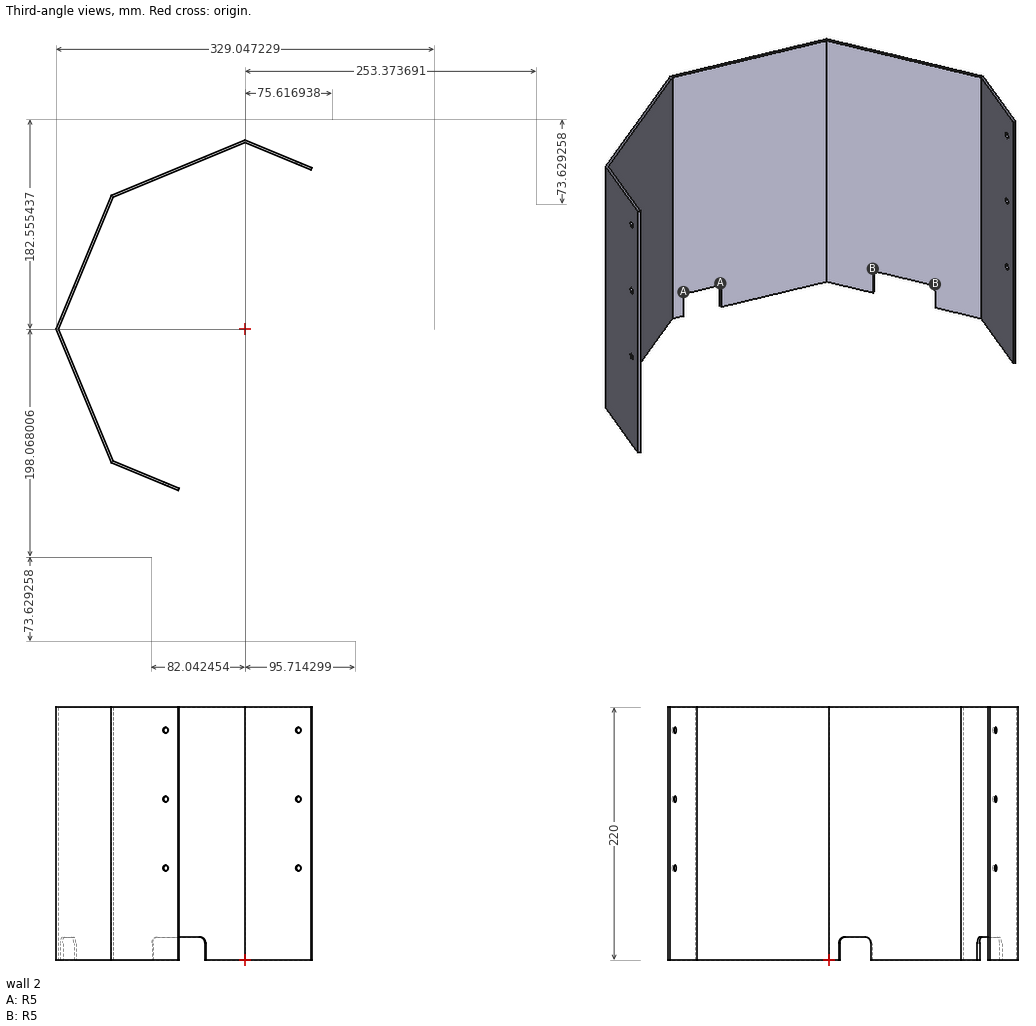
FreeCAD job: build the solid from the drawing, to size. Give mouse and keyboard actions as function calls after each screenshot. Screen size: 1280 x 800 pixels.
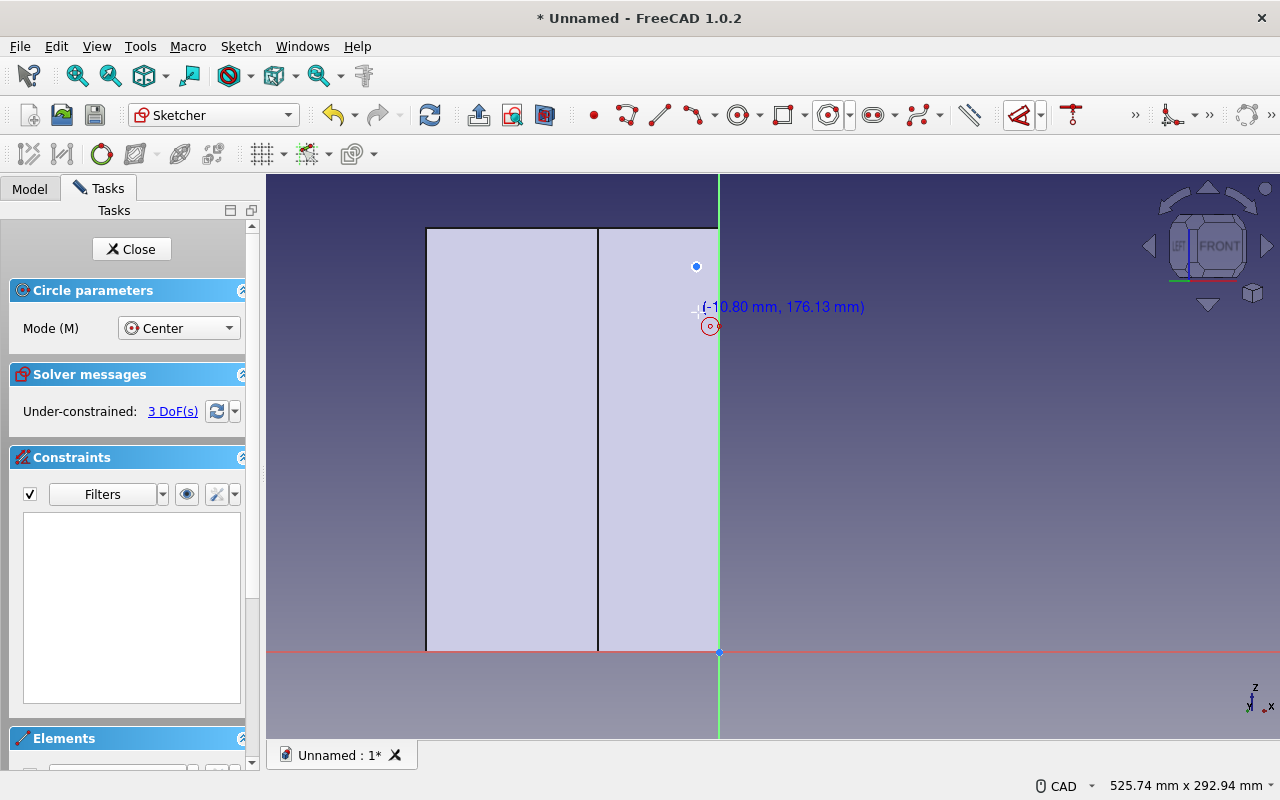
click(696, 382)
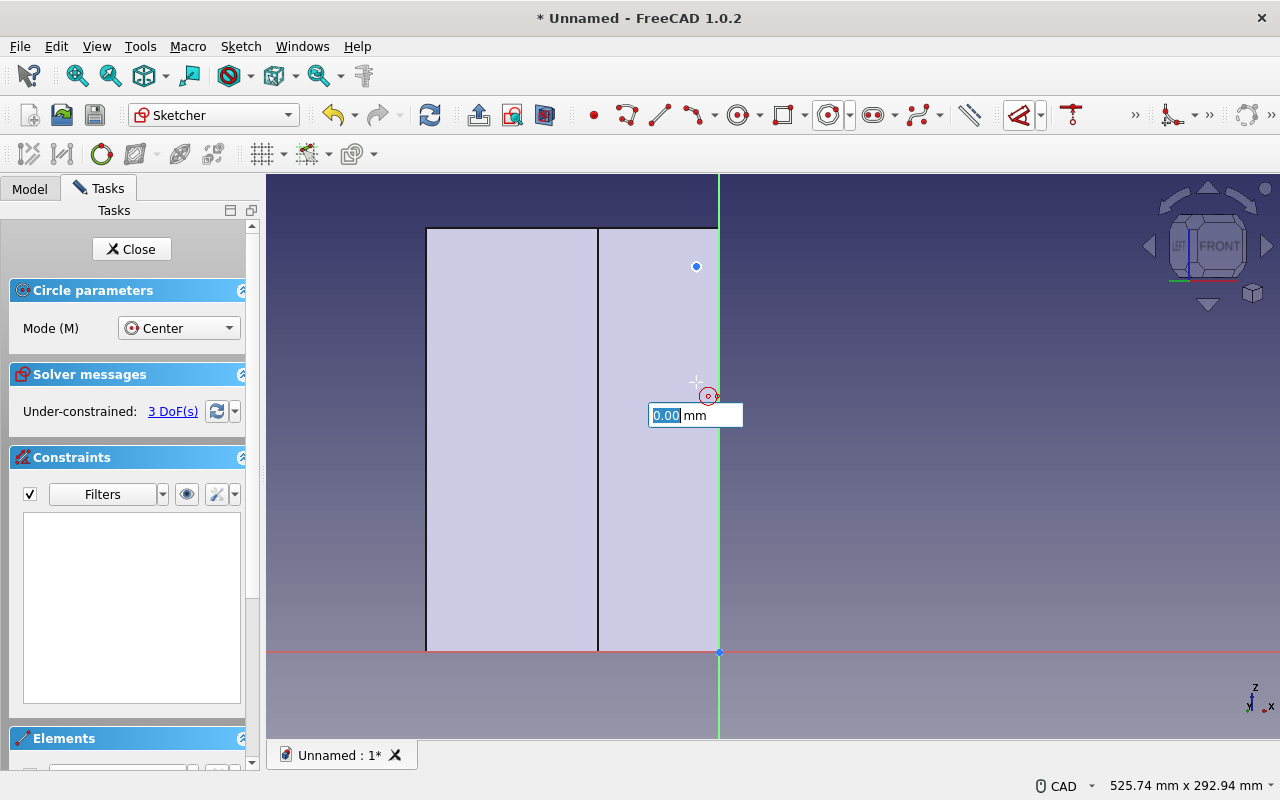
scroll(699, 379, up, 6)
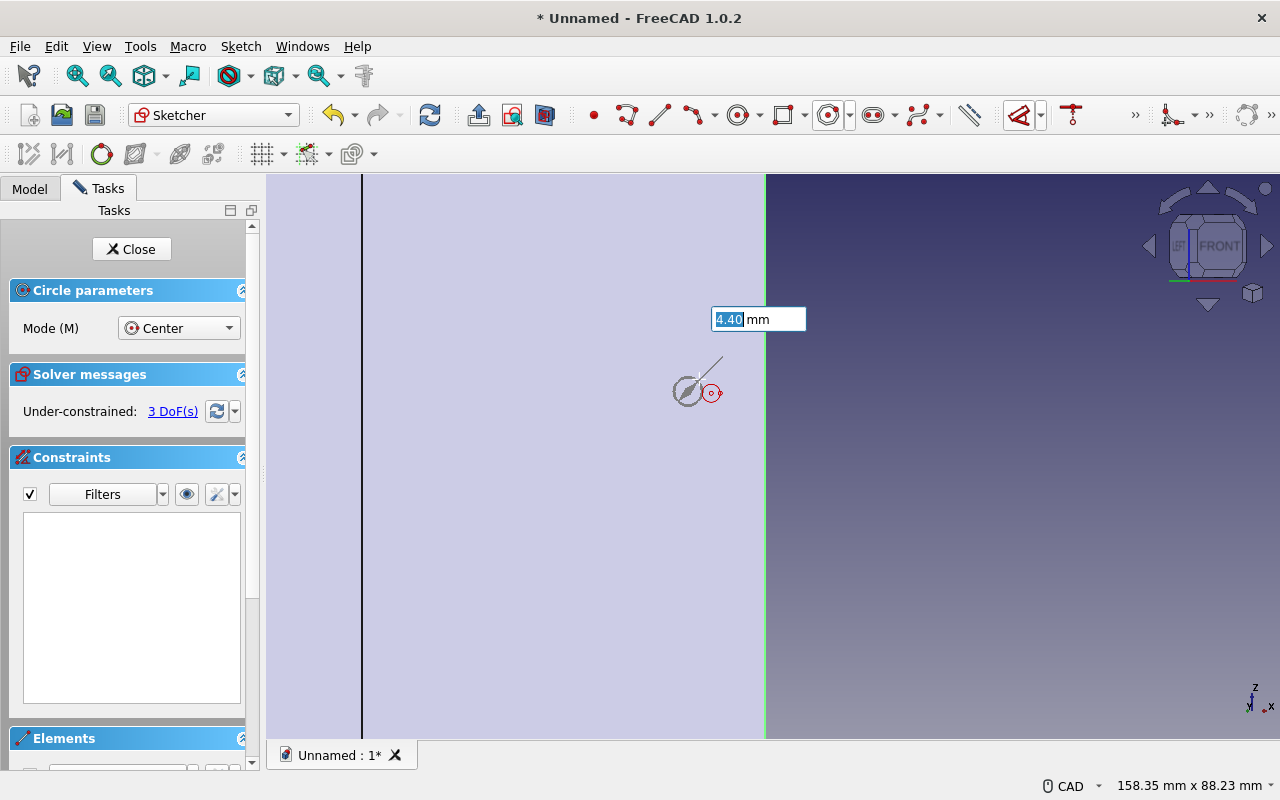
click(699, 377)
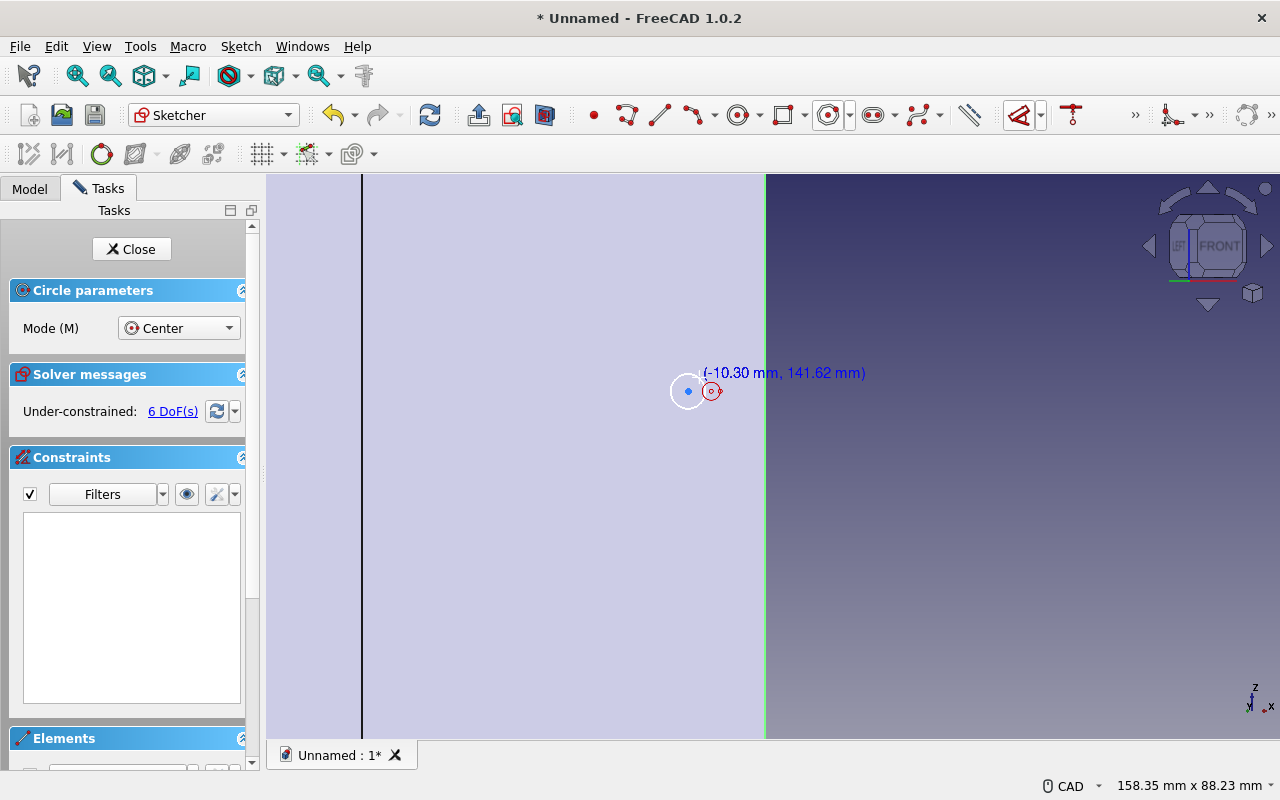
scroll(698, 379, down, 6)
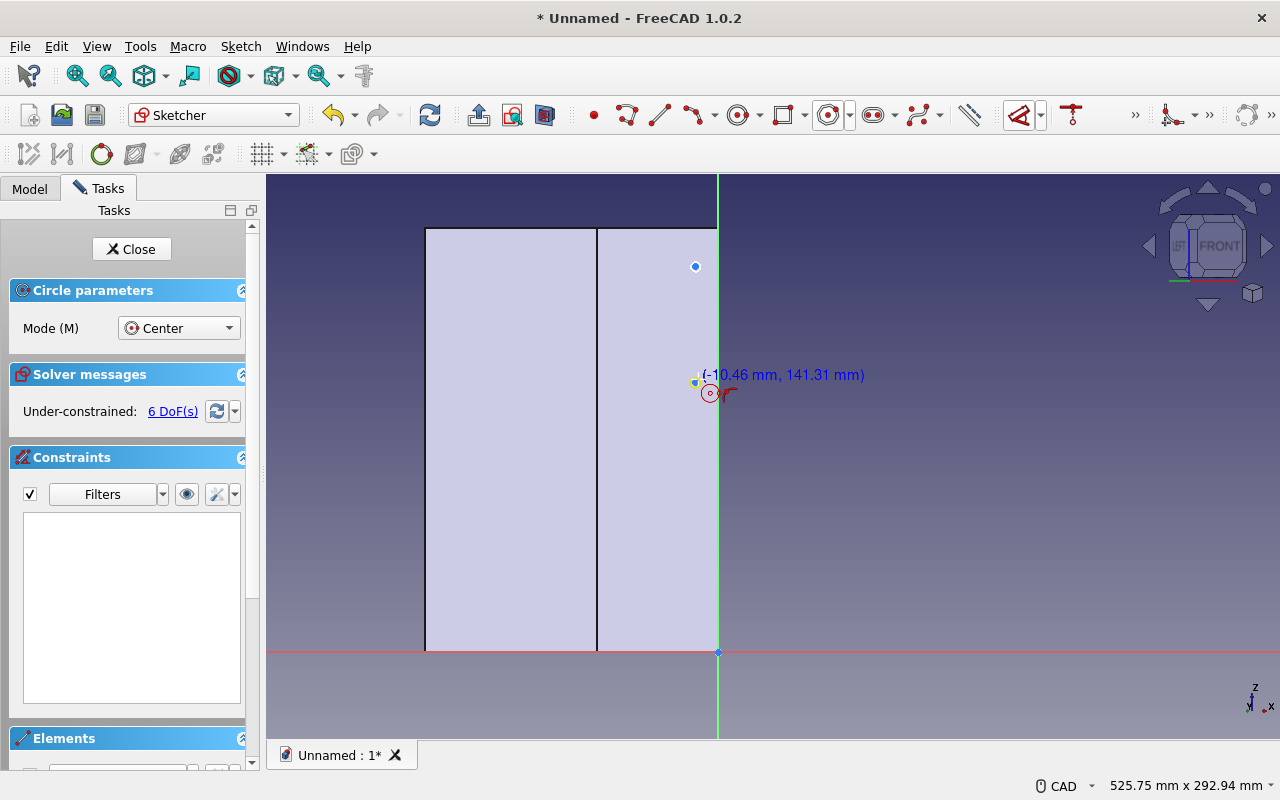
scroll(695, 498, up, 8)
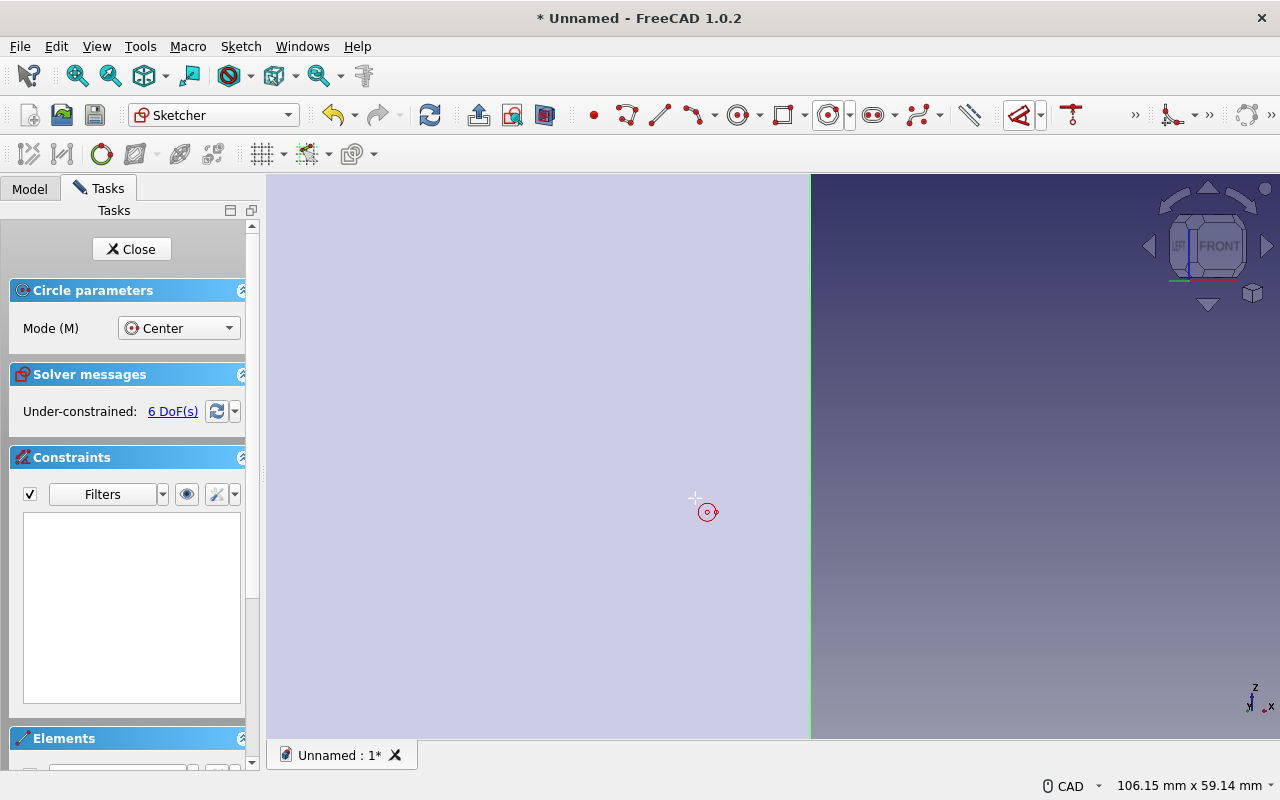
scroll(695, 498, down, 8)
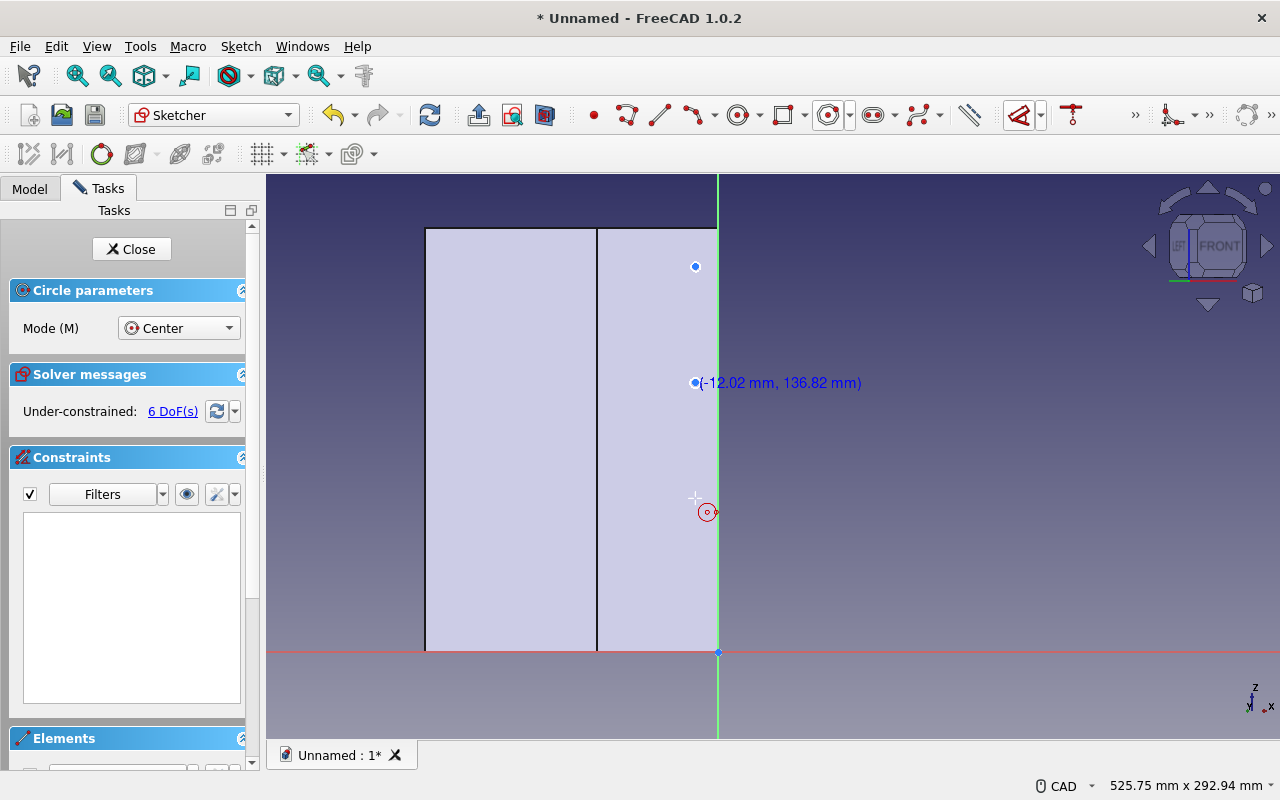
click(695, 498)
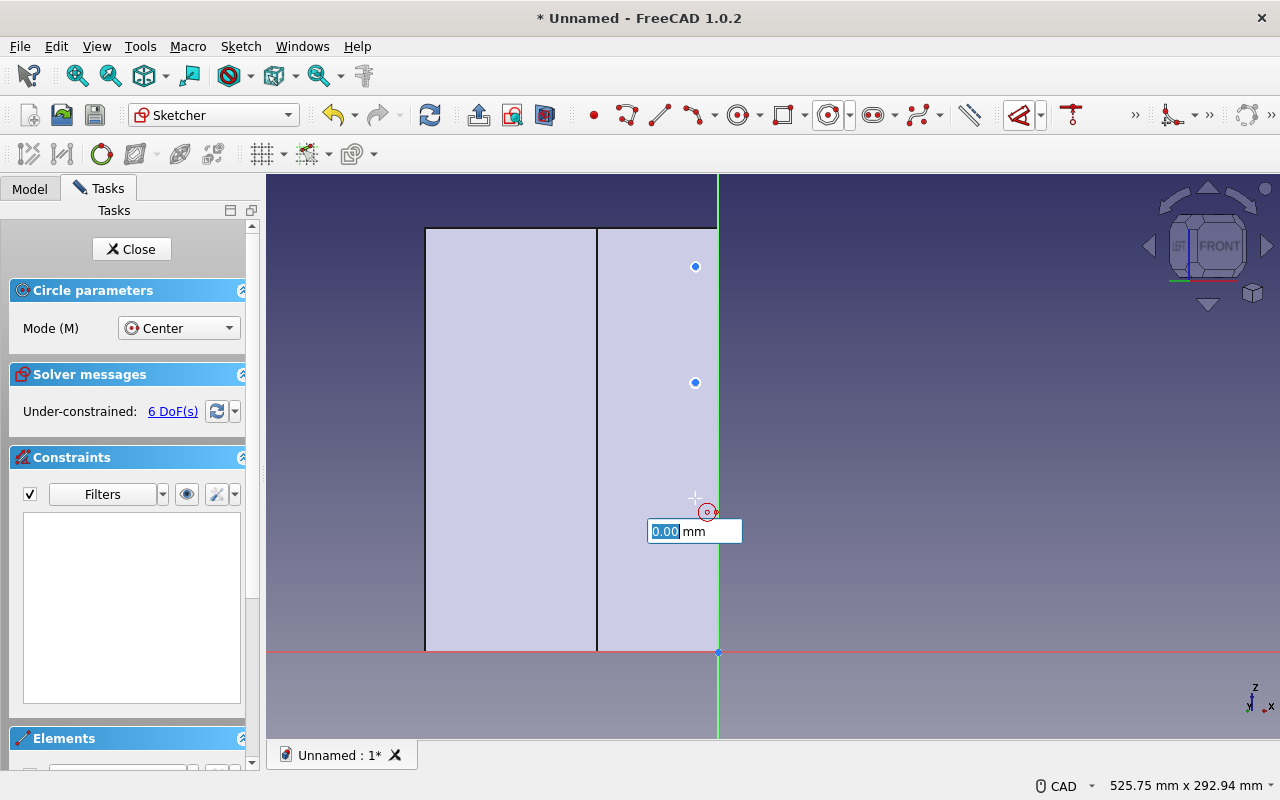
scroll(699, 494, up, 6)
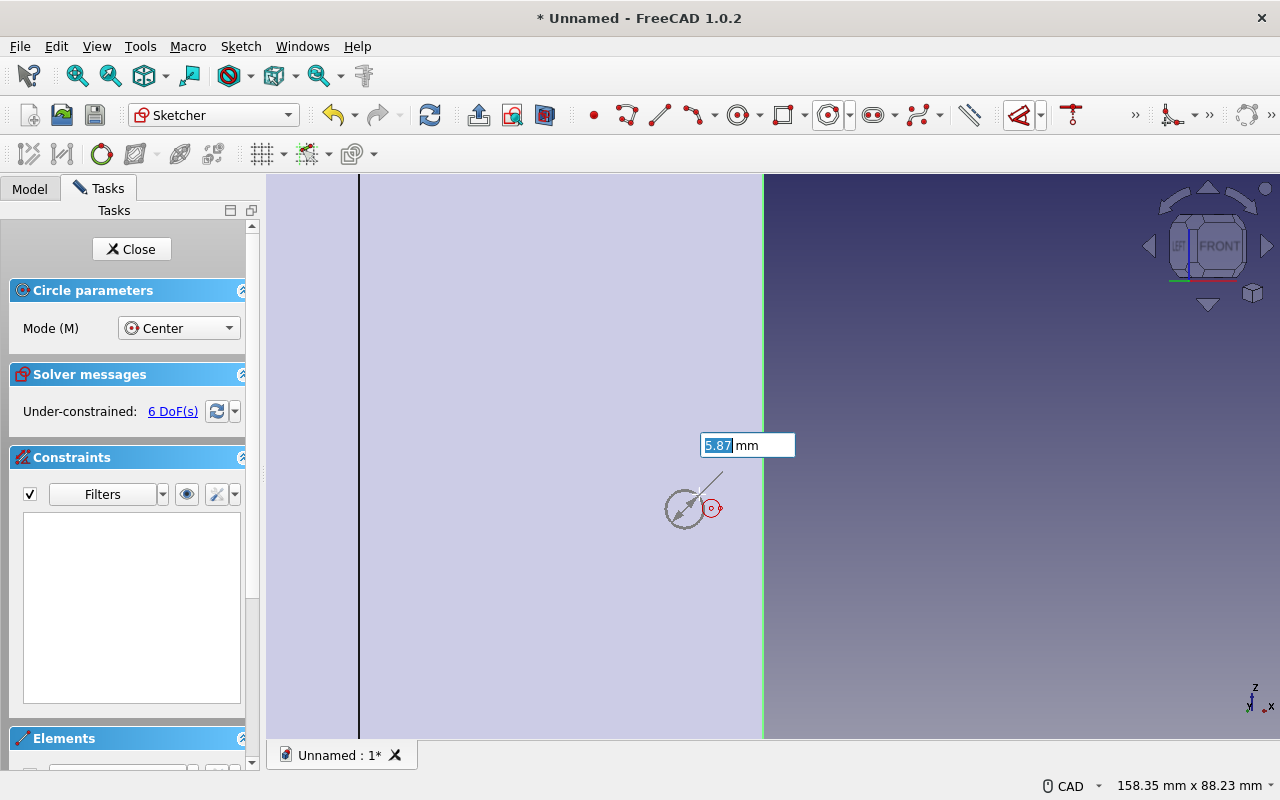
click(697, 494)
key(Escape)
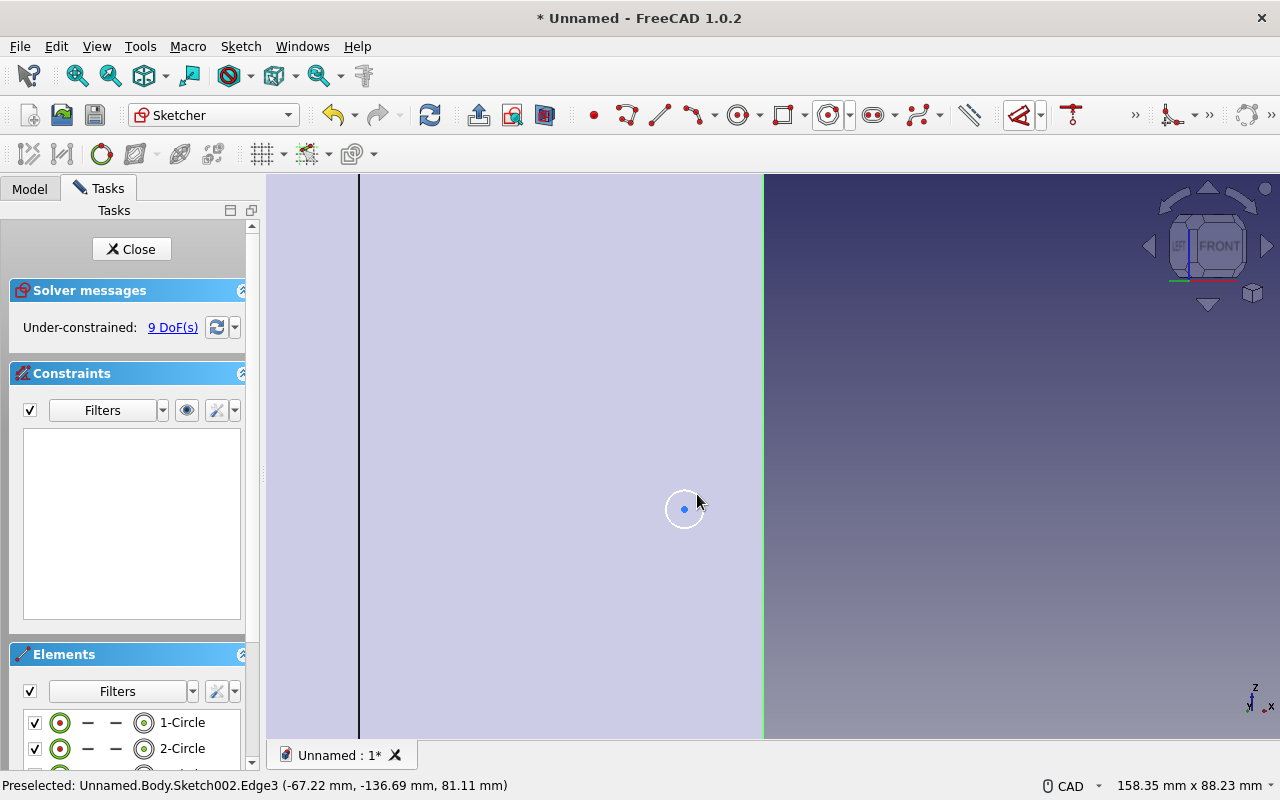
scroll(699, 494, down, 6)